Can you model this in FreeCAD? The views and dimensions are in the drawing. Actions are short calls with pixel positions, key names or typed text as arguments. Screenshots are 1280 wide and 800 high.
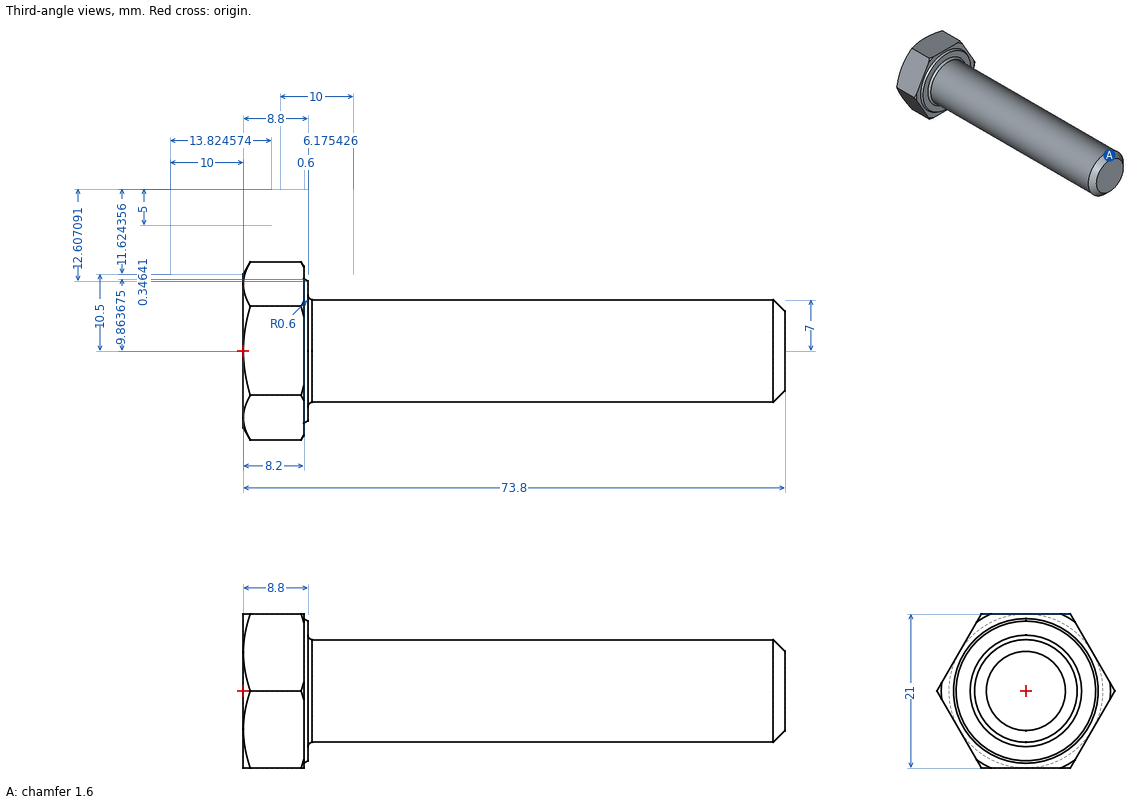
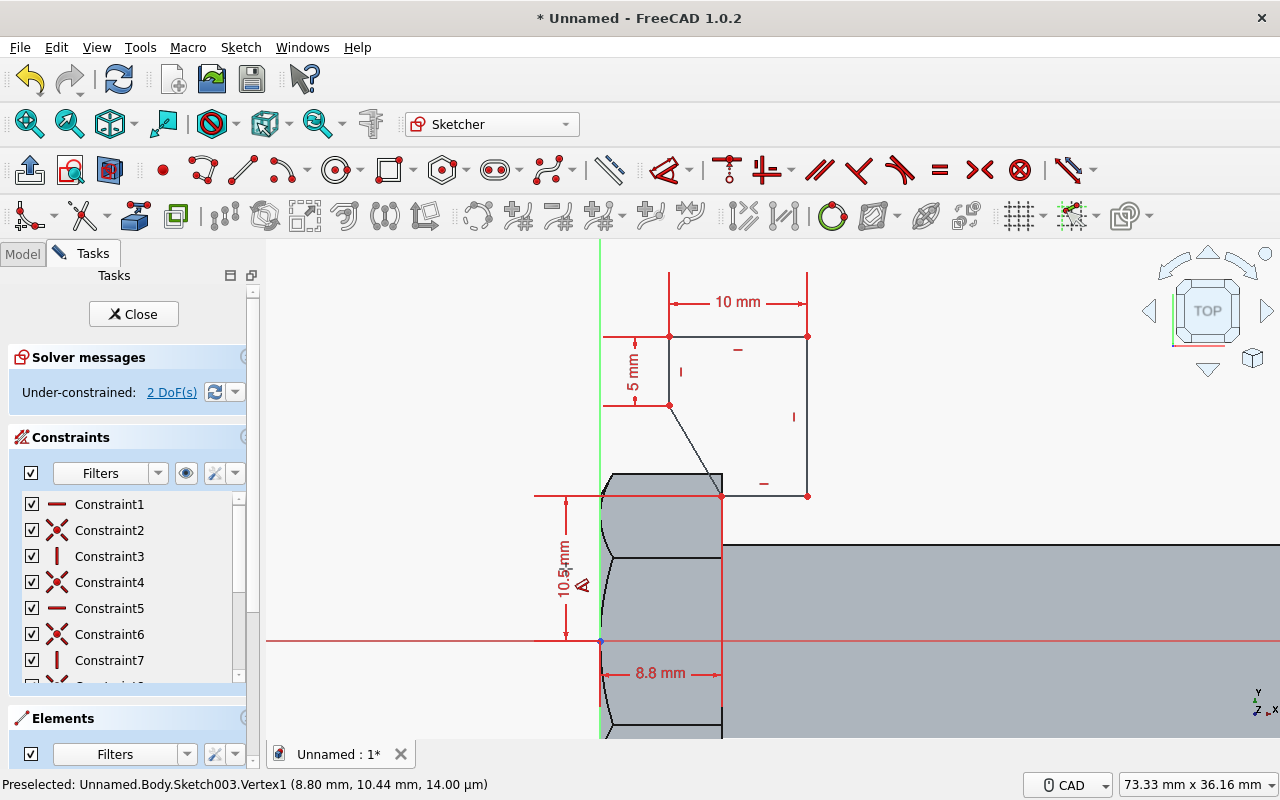
click(747, 496)
click(765, 530)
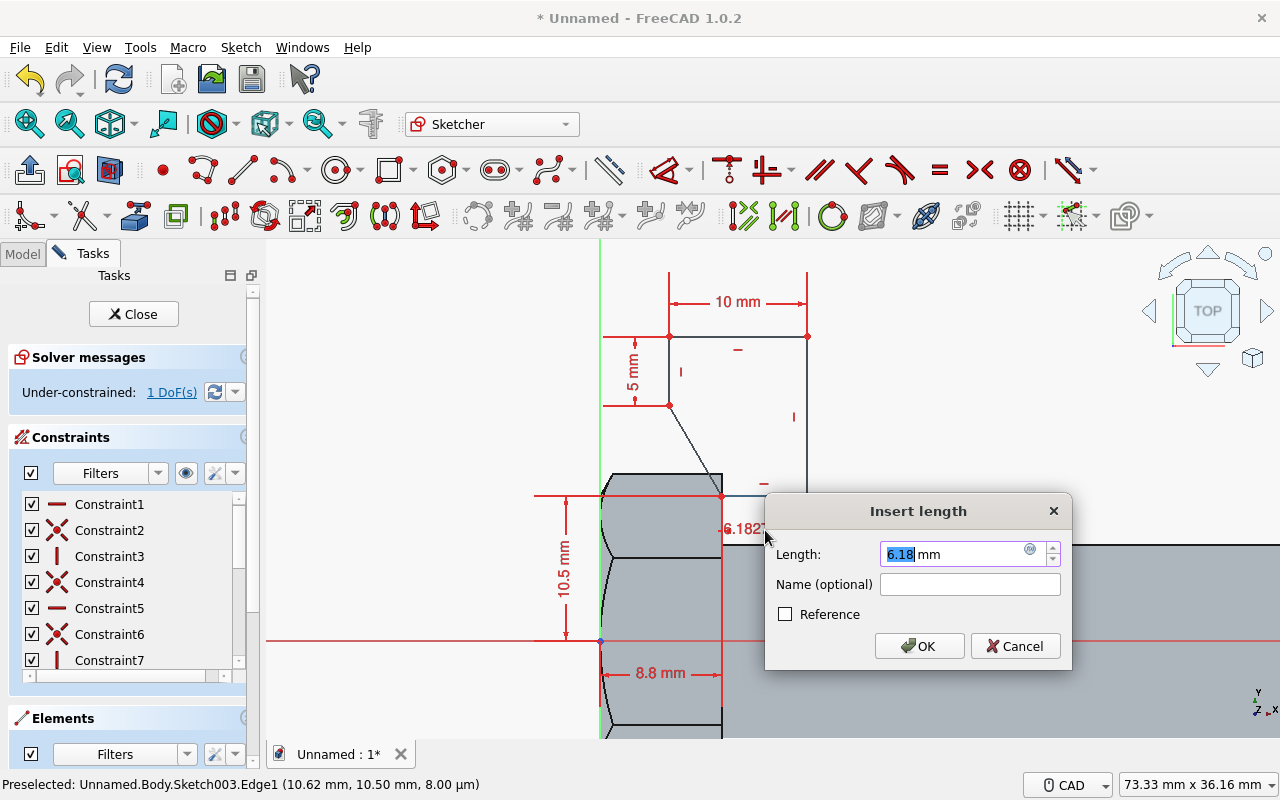
text(6.175426)
key(Return)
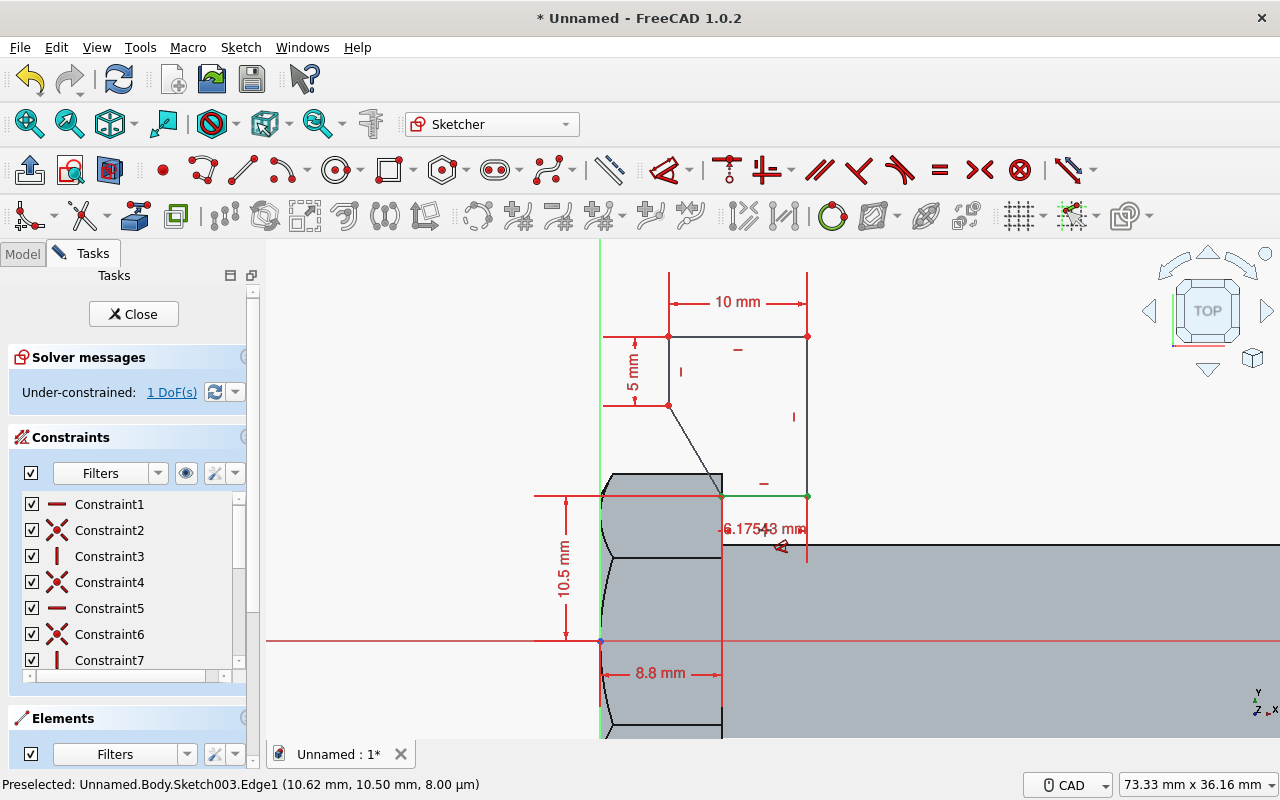
click(807, 448)
click(841, 417)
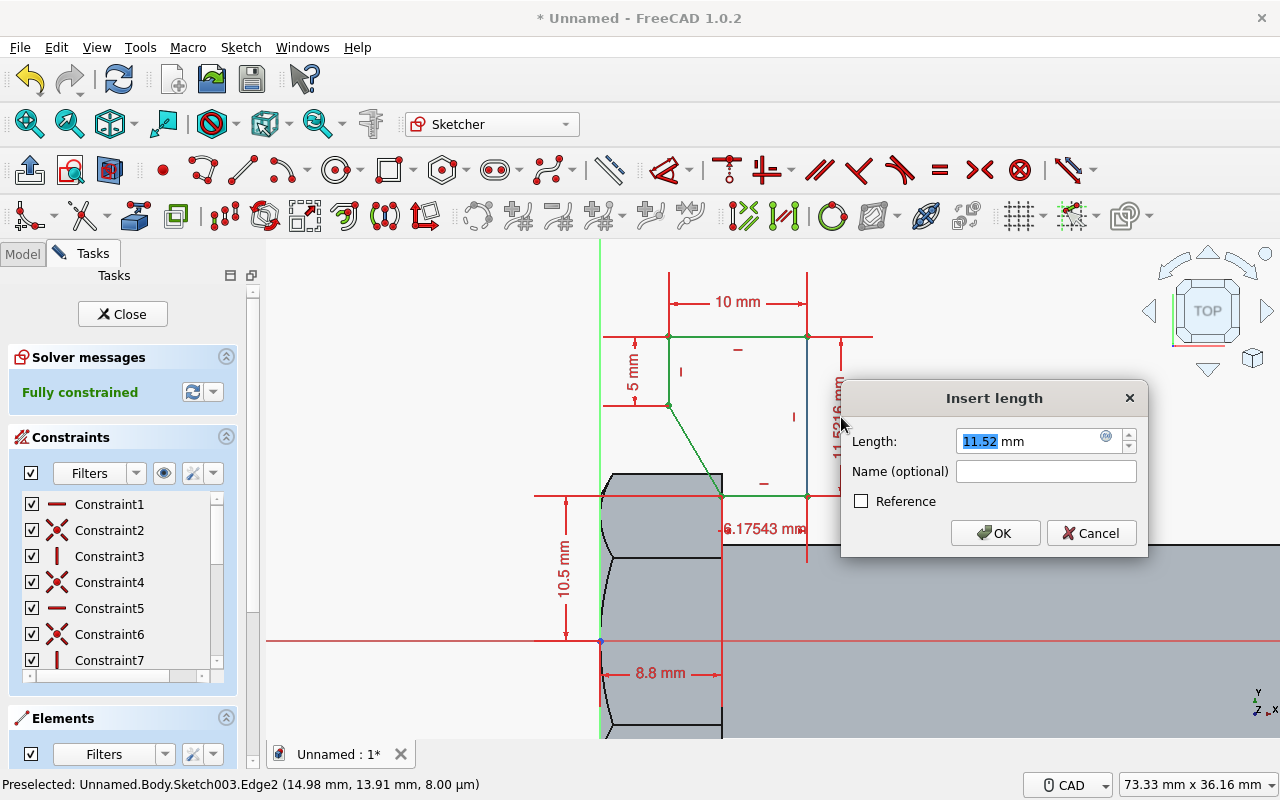
text(11.624356)
key(Return)
key(Escape)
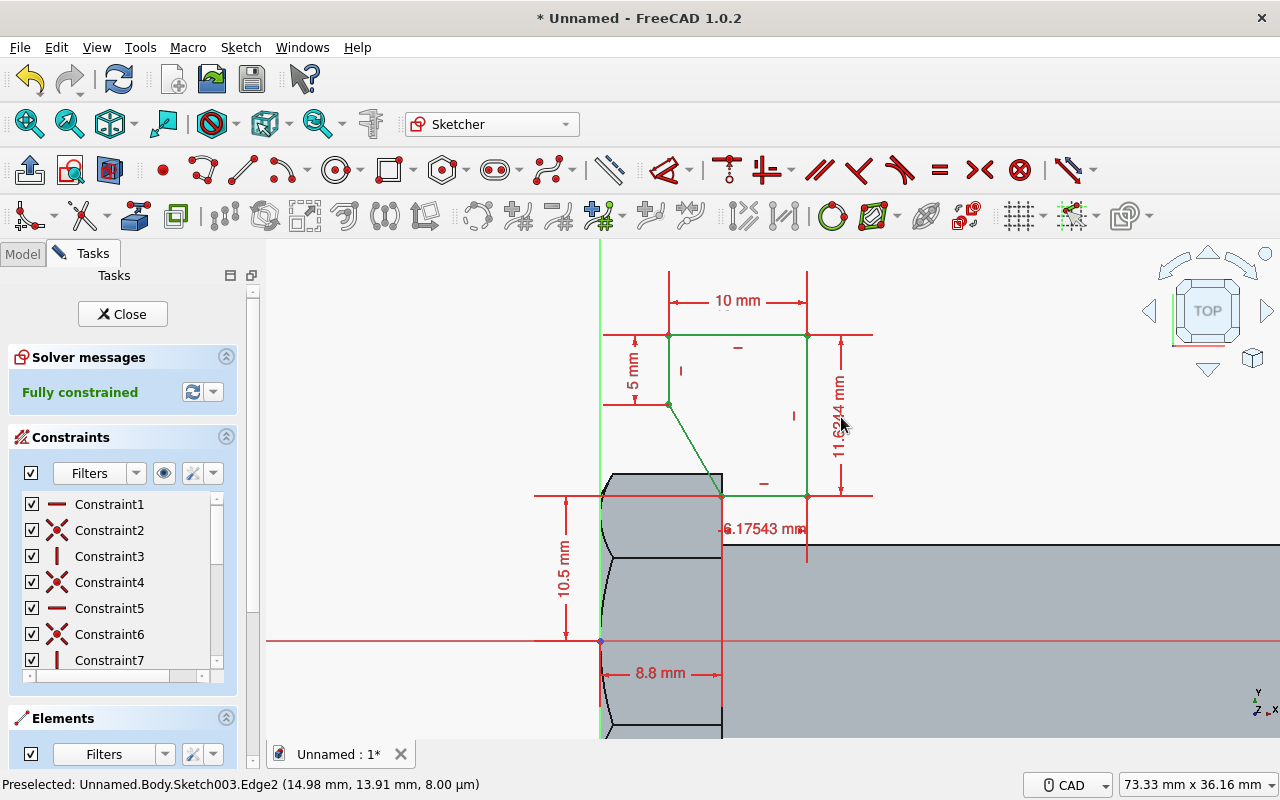
click(123, 314)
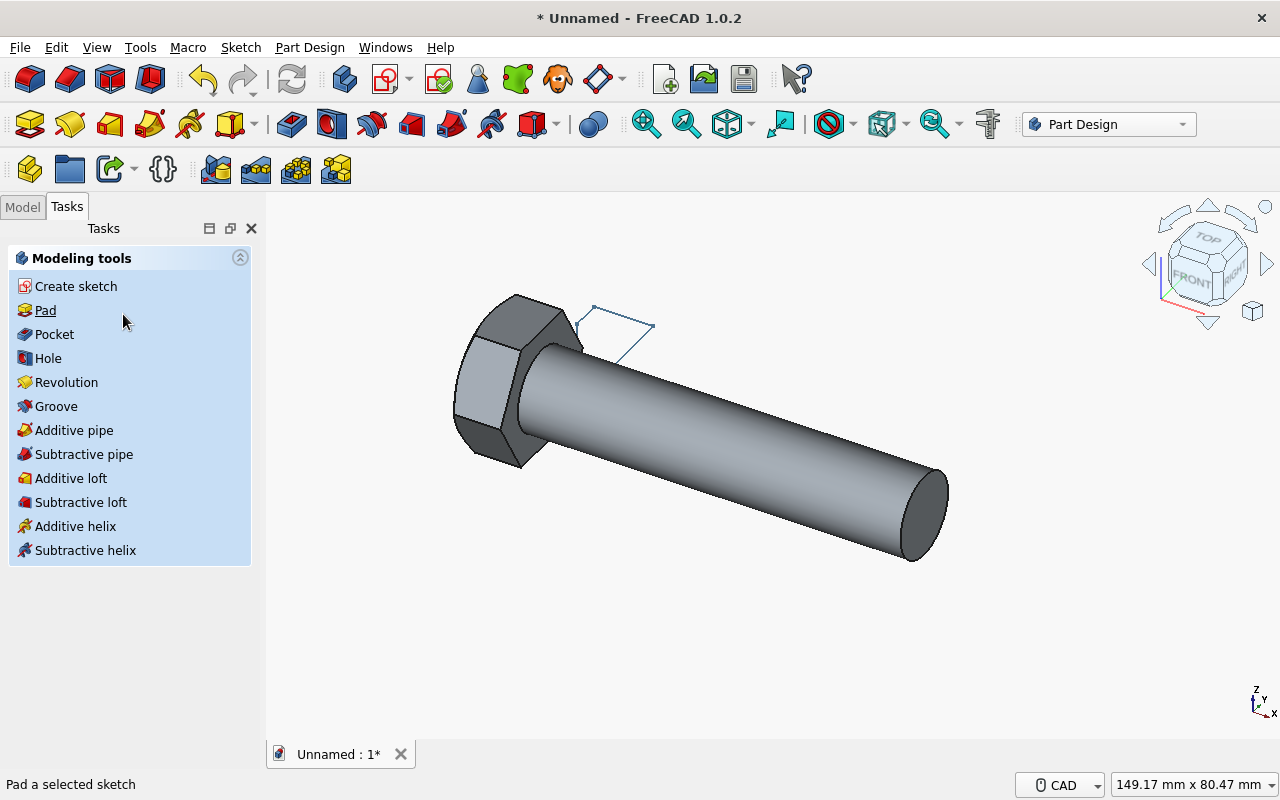
click(372, 124)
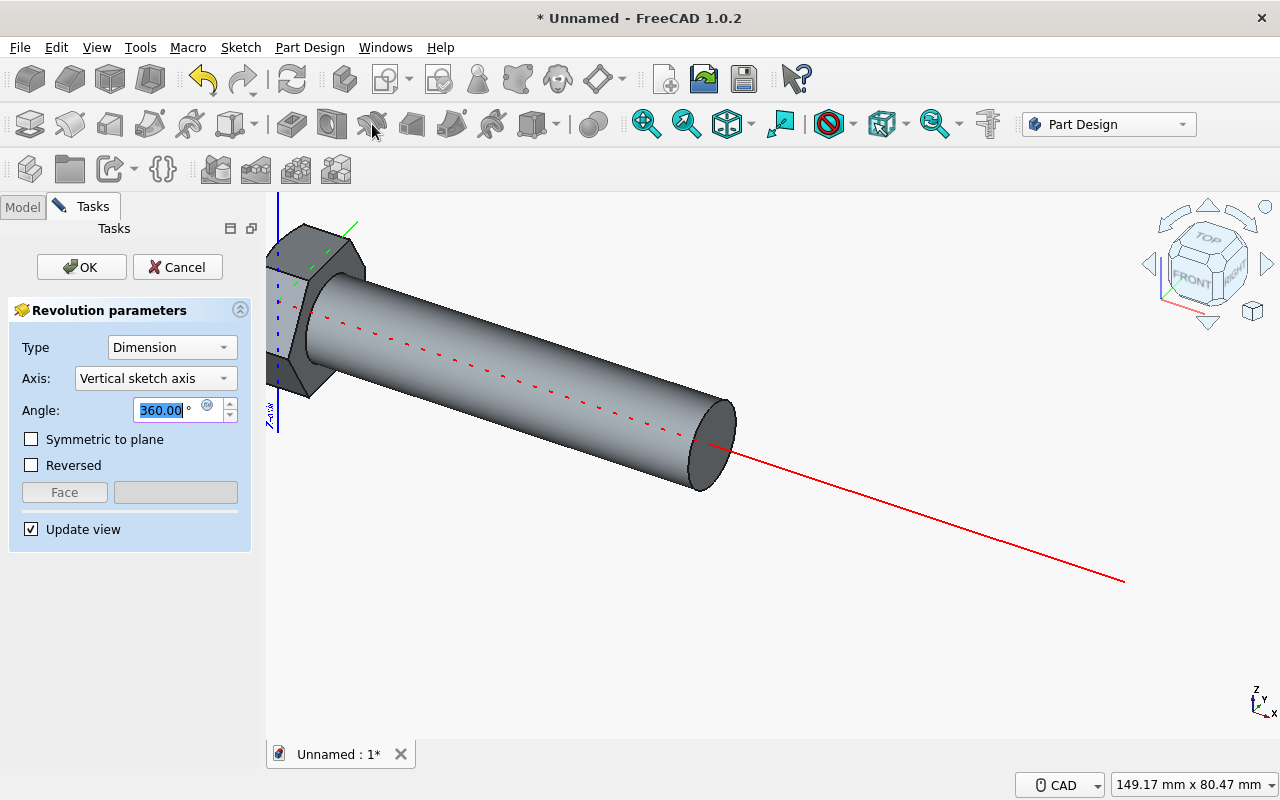
click(156, 378)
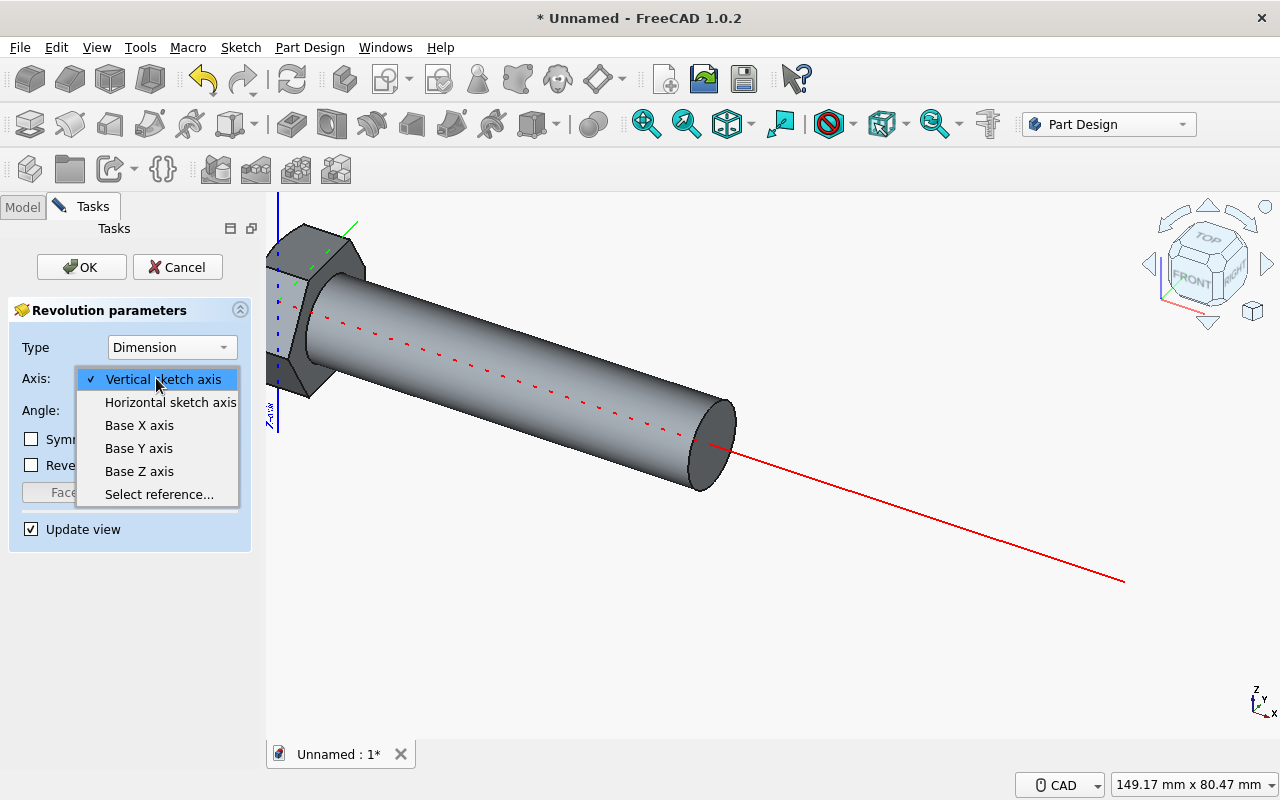
click(156, 402)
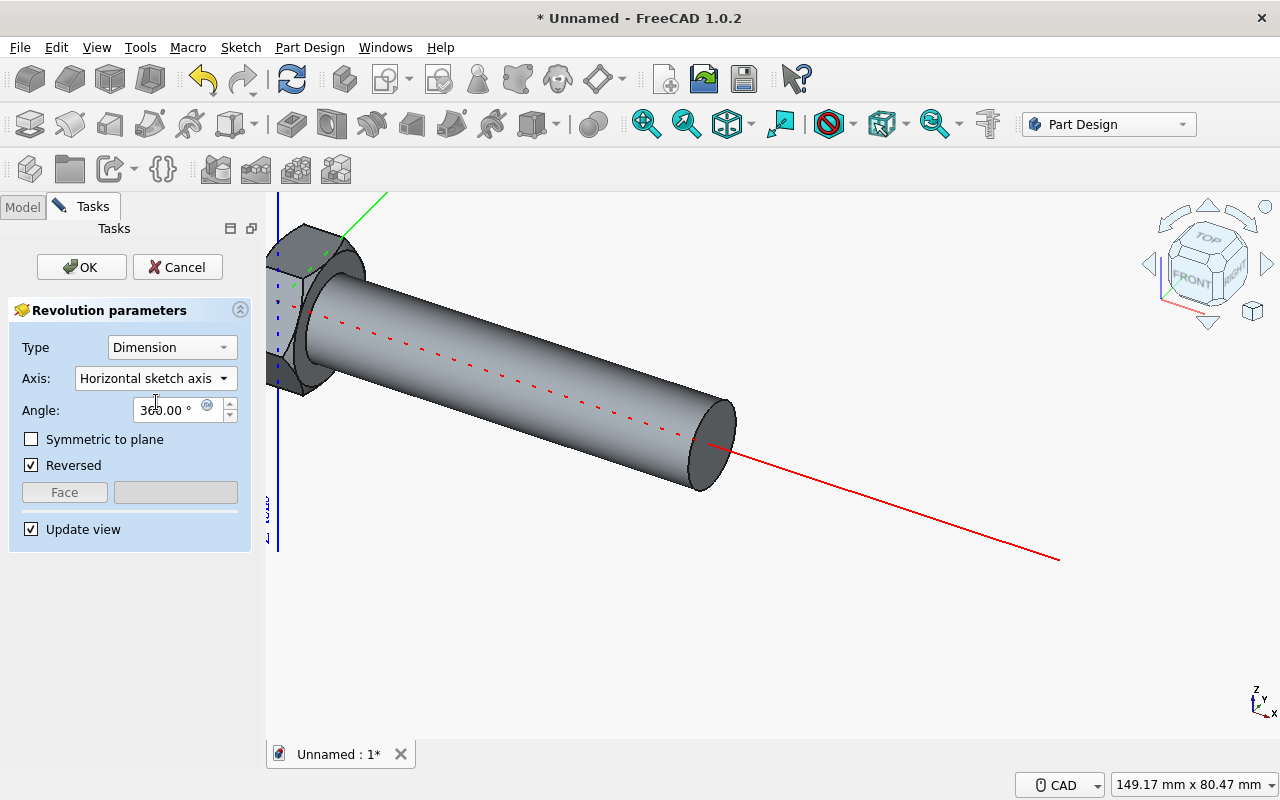
click(82, 267)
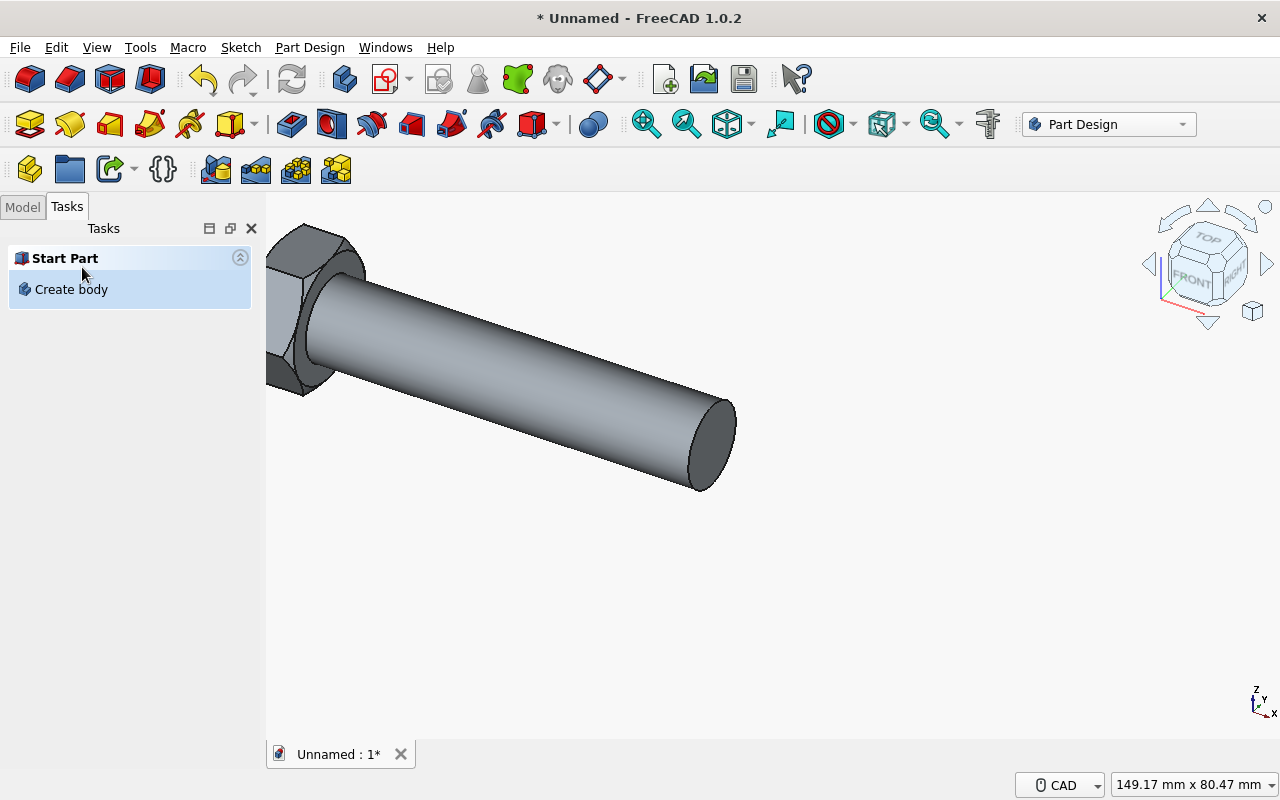
click(648, 124)